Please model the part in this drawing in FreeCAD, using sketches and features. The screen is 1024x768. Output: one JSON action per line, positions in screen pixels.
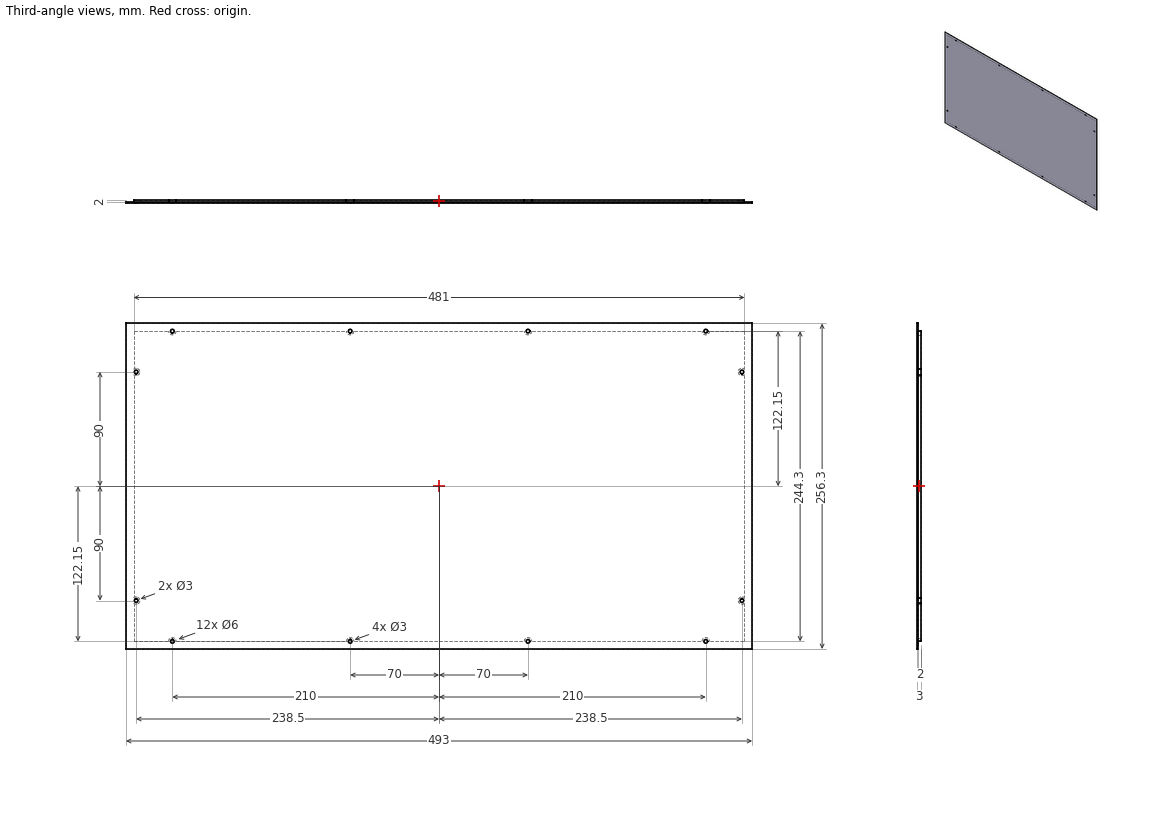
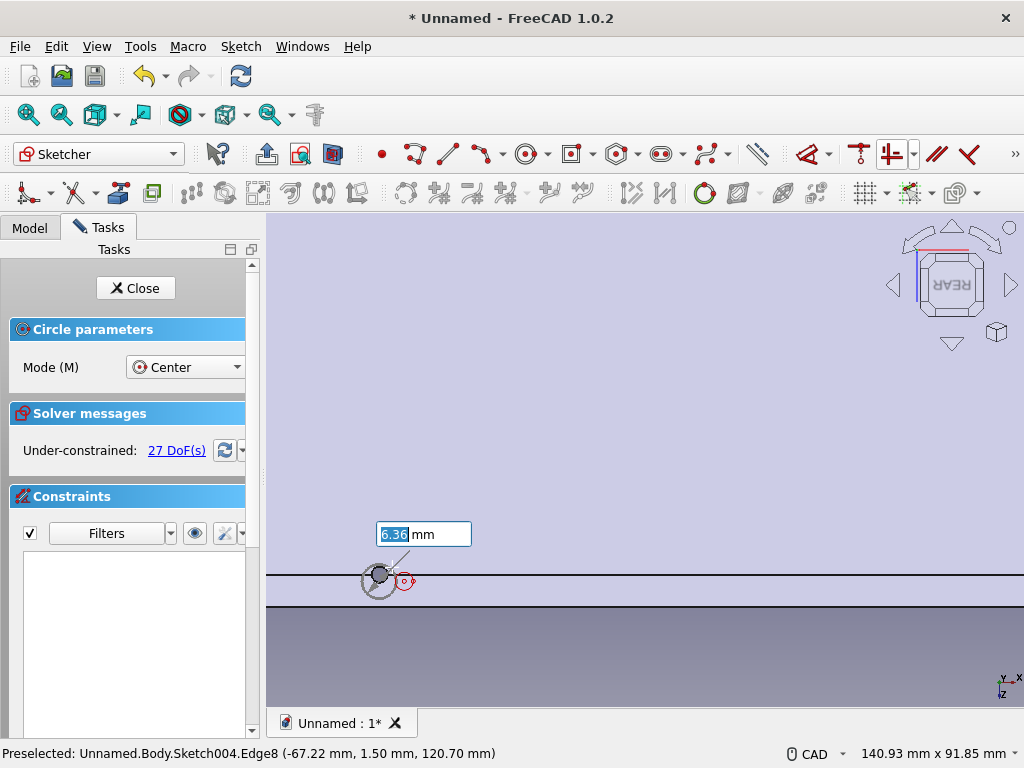
{"action": "left_click", "coordinate": [391, 563]}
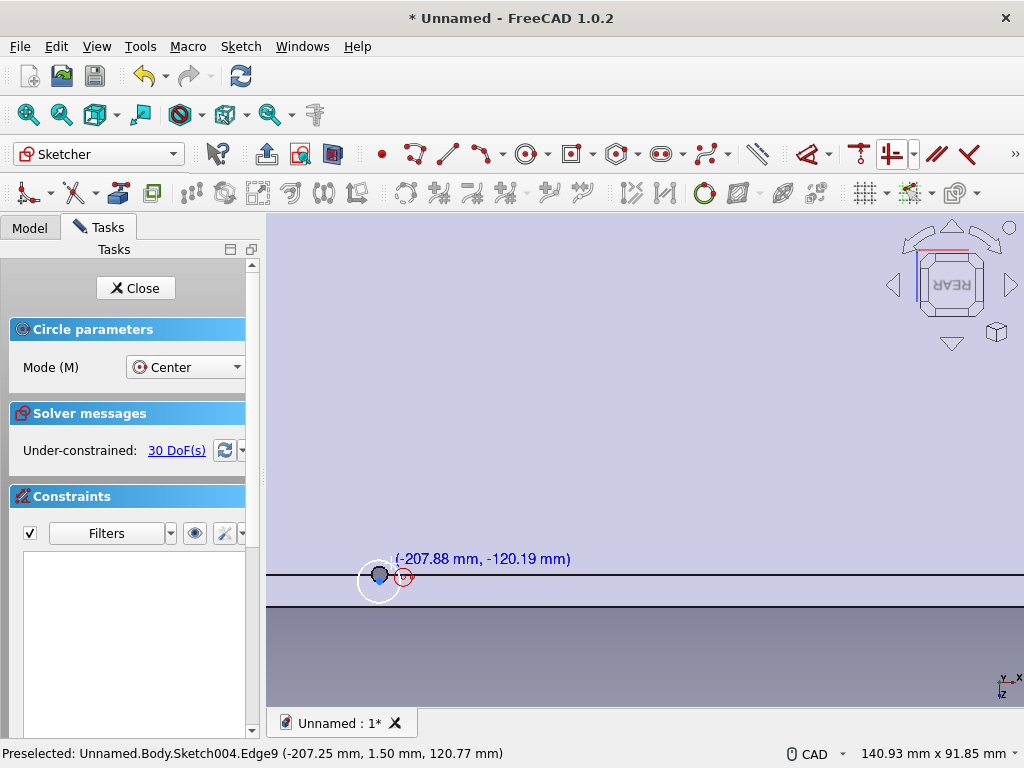
{"action": "scroll", "coordinate": [392, 567], "scroll_direction": "down", "scroll_amount": 9}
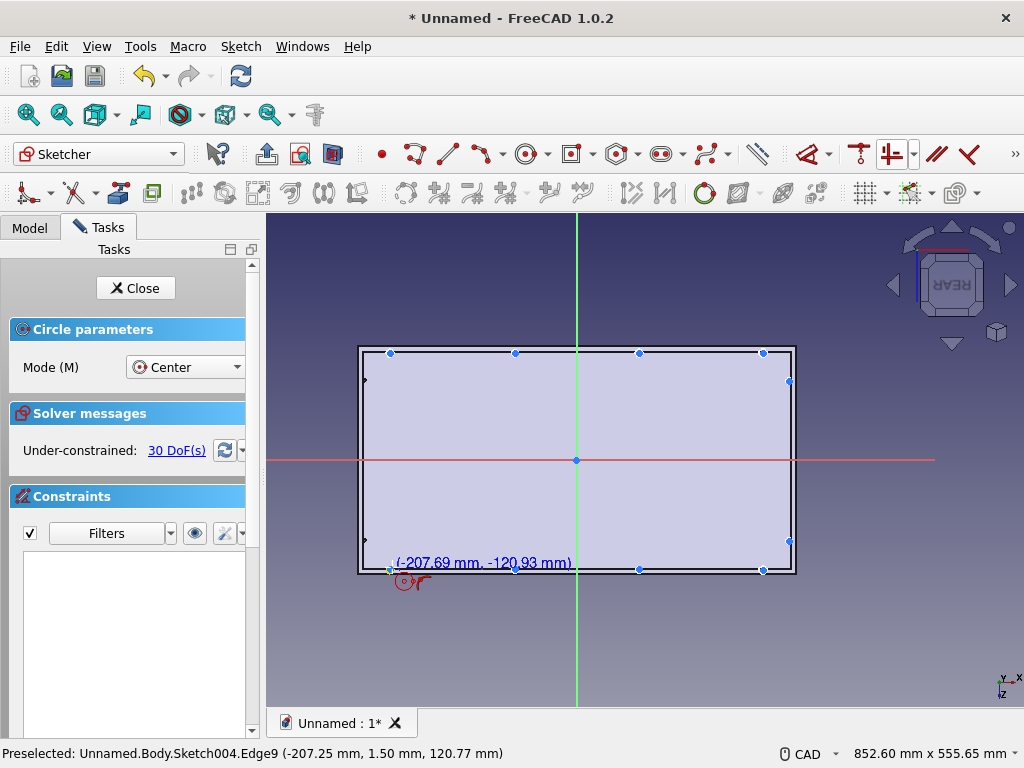
{"action": "scroll", "coordinate": [365, 540], "scroll_direction": "up", "scroll_amount": 11}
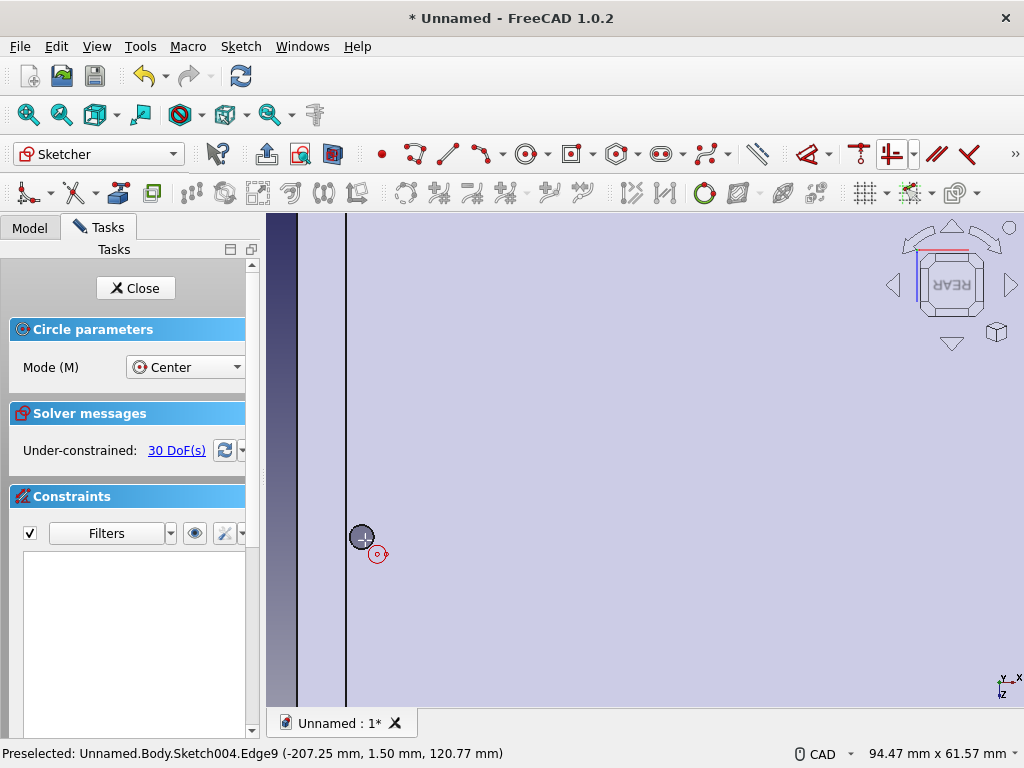
{"action": "scroll", "coordinate": [365, 540], "scroll_direction": "down", "scroll_amount": 11}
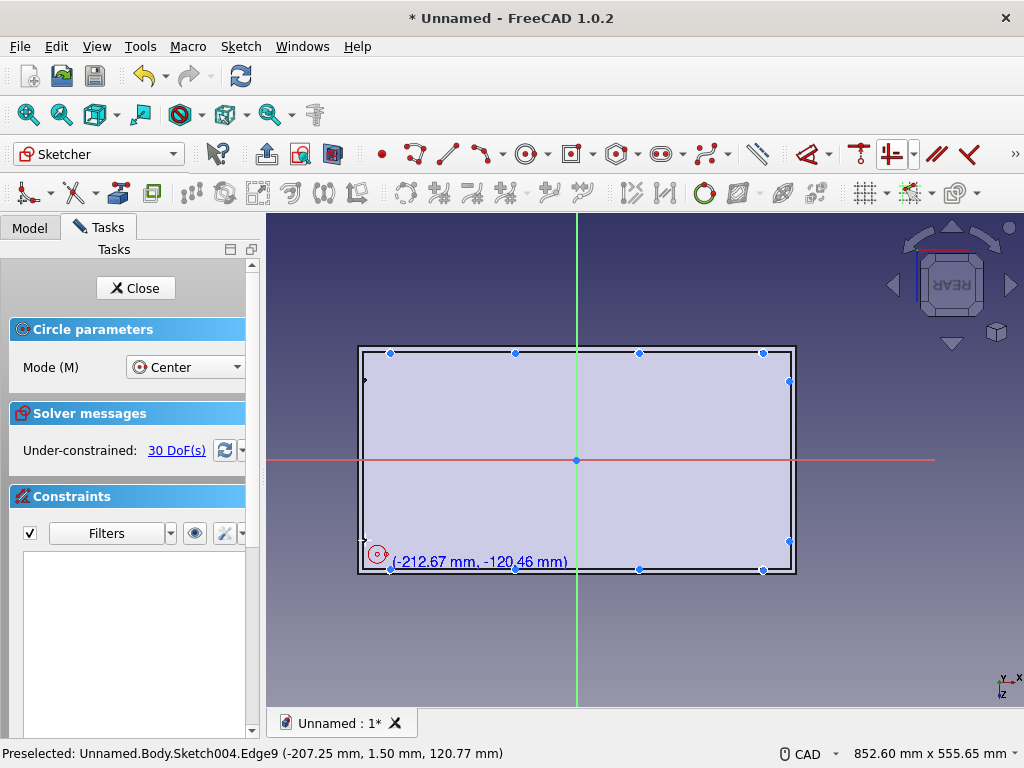
{"action": "left_click", "coordinate": [365, 540]}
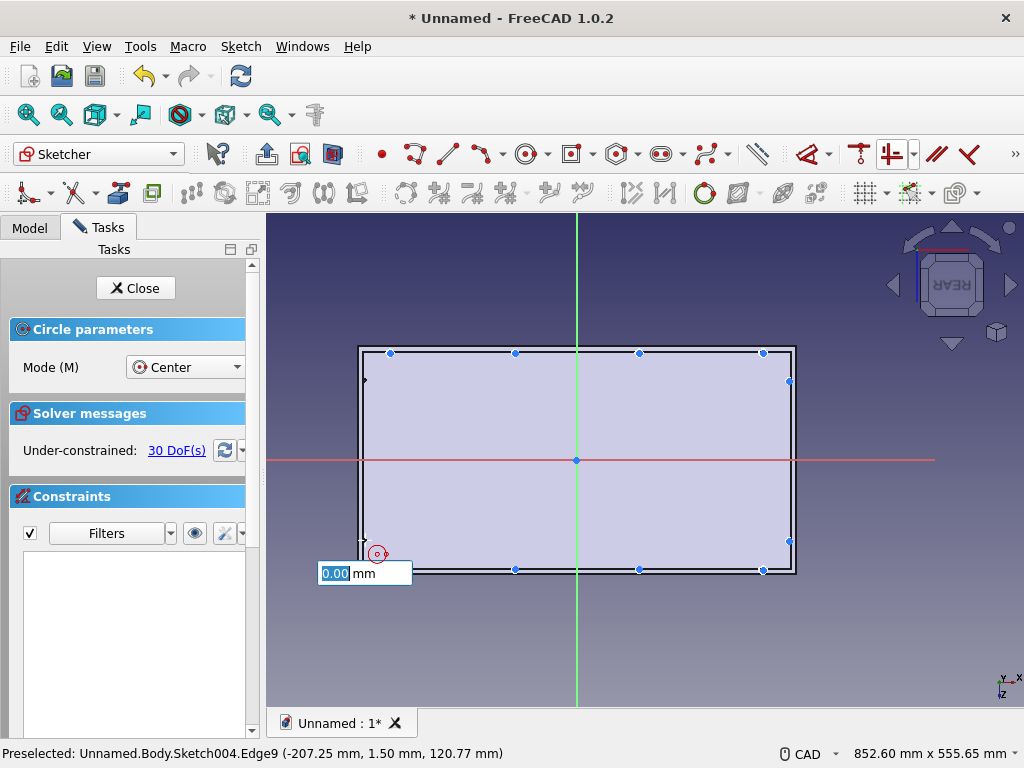
{"action": "scroll", "coordinate": [367, 538], "scroll_direction": "up", "scroll_amount": 9}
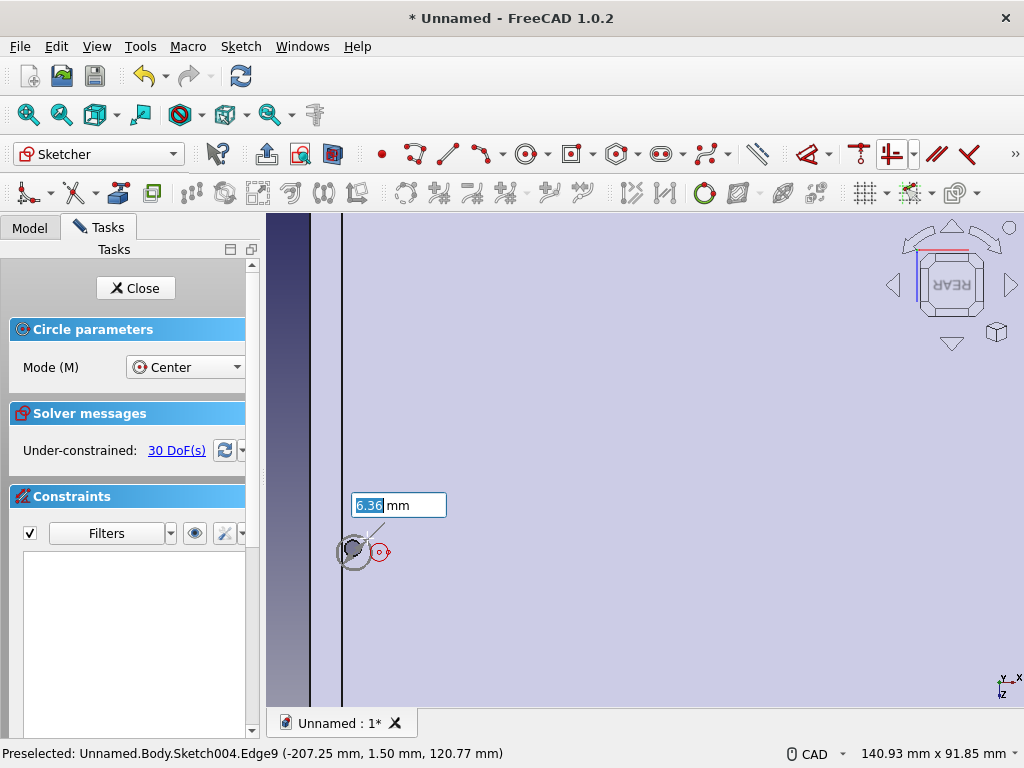
{"action": "left_click", "coordinate": [364, 537]}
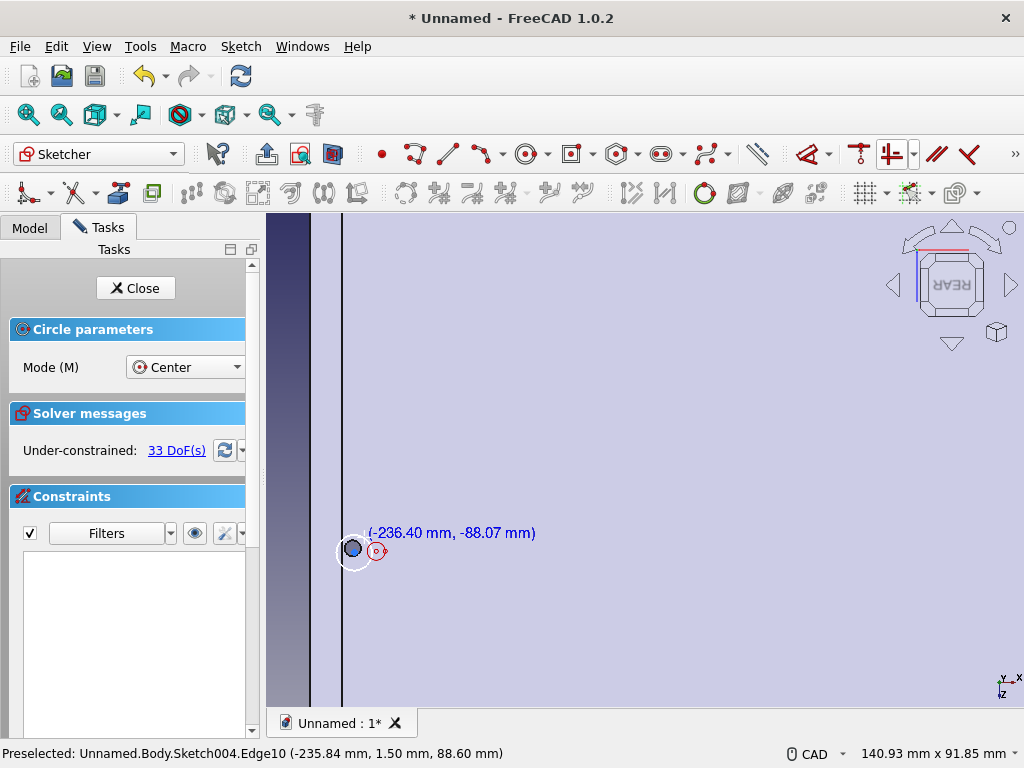
{"action": "scroll", "coordinate": [367, 538], "scroll_direction": "down", "scroll_amount": 9}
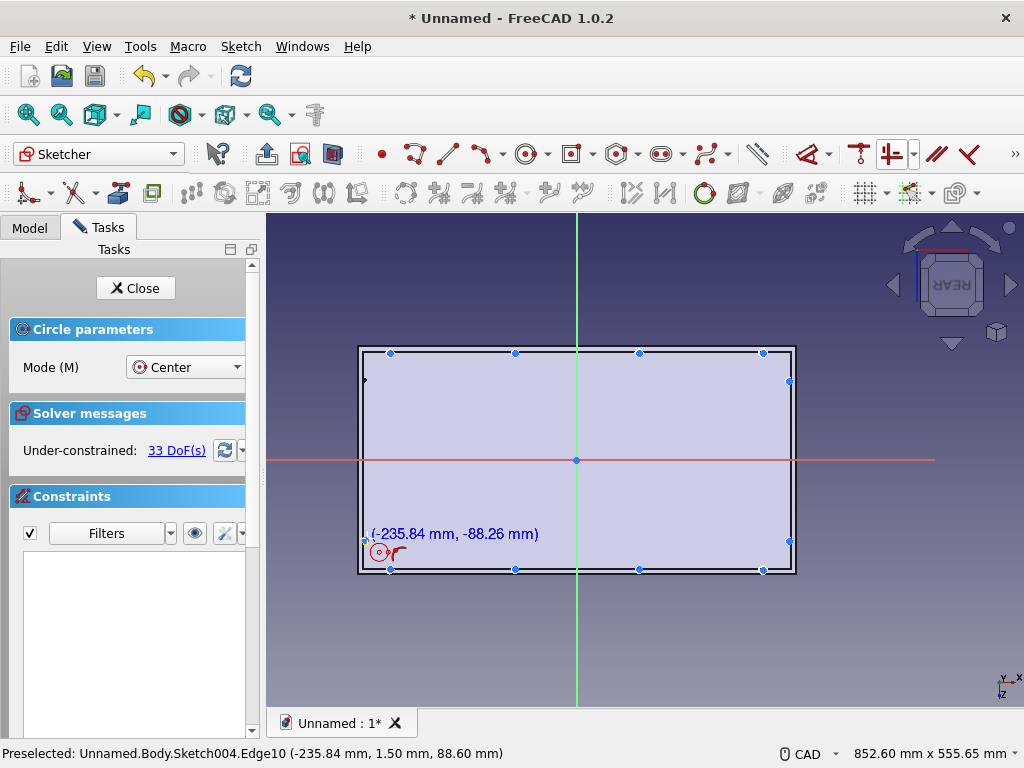
{"action": "scroll", "coordinate": [365, 380], "scroll_direction": "up", "scroll_amount": 11}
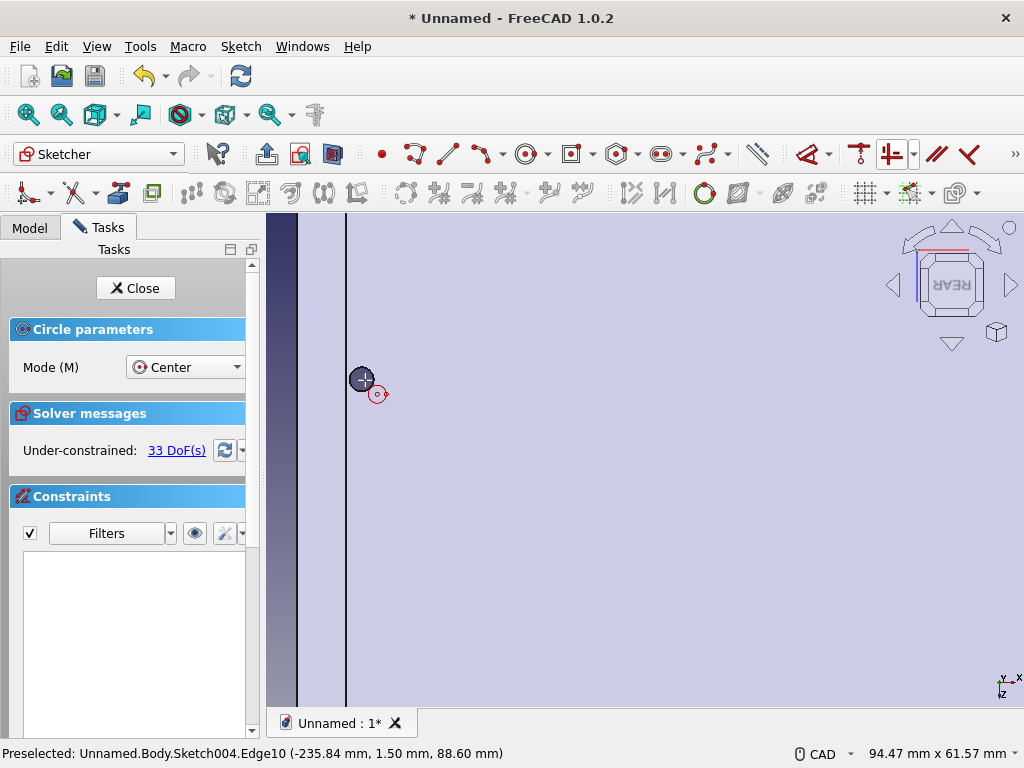
{"action": "scroll", "coordinate": [365, 380], "scroll_direction": "down", "scroll_amount": 11}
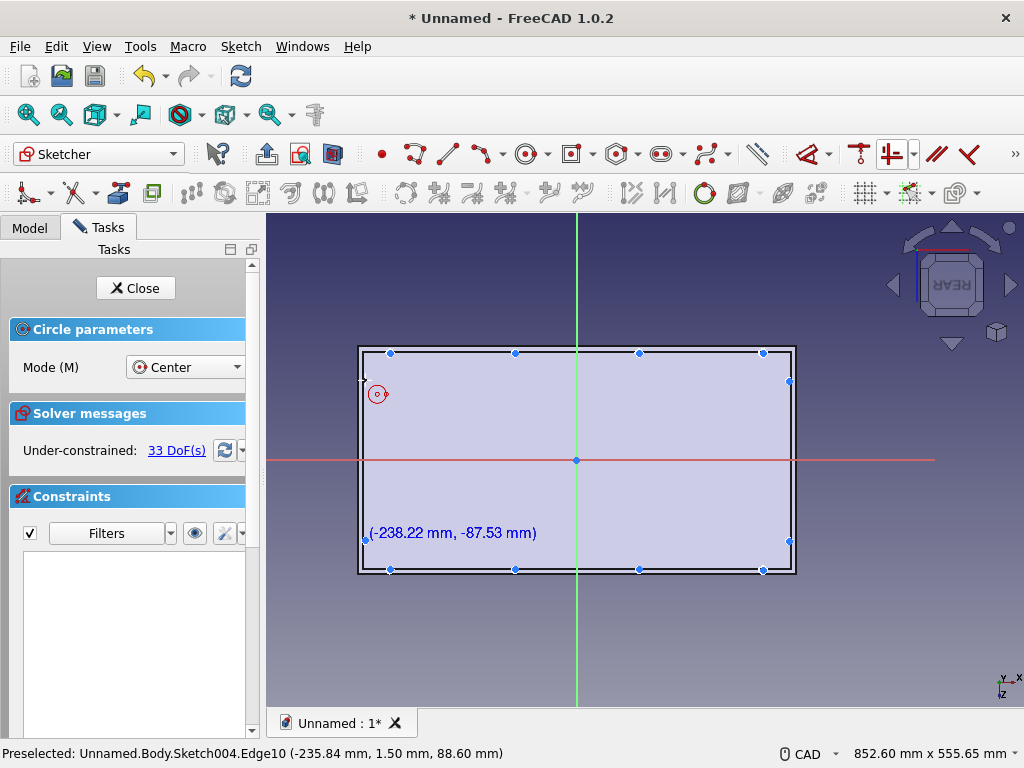
{"action": "left_click", "coordinate": [365, 380]}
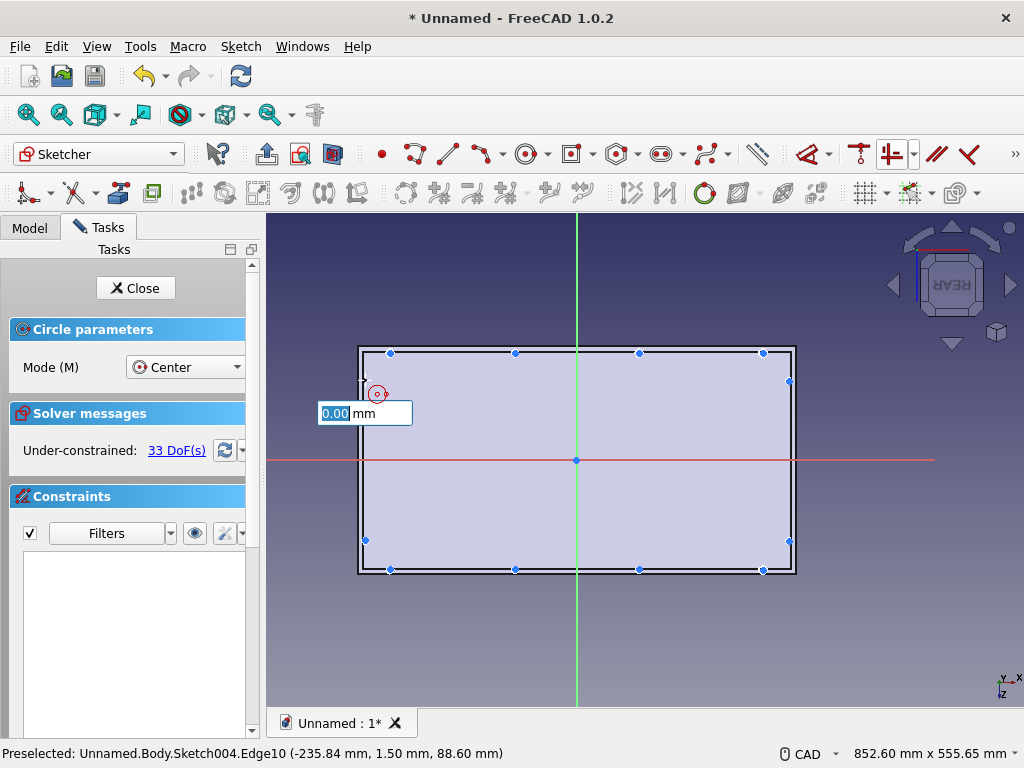
{"action": "scroll", "coordinate": [367, 378], "scroll_direction": "up", "scroll_amount": 9}